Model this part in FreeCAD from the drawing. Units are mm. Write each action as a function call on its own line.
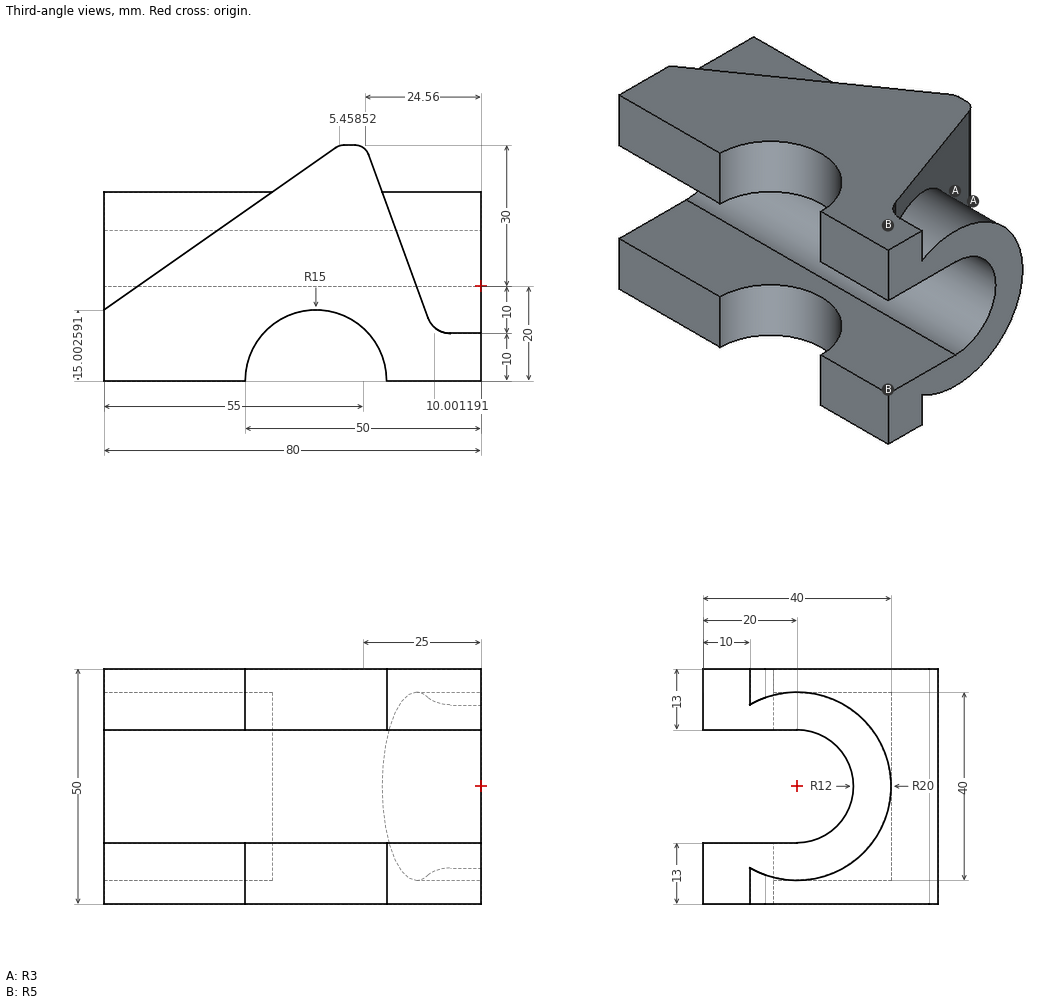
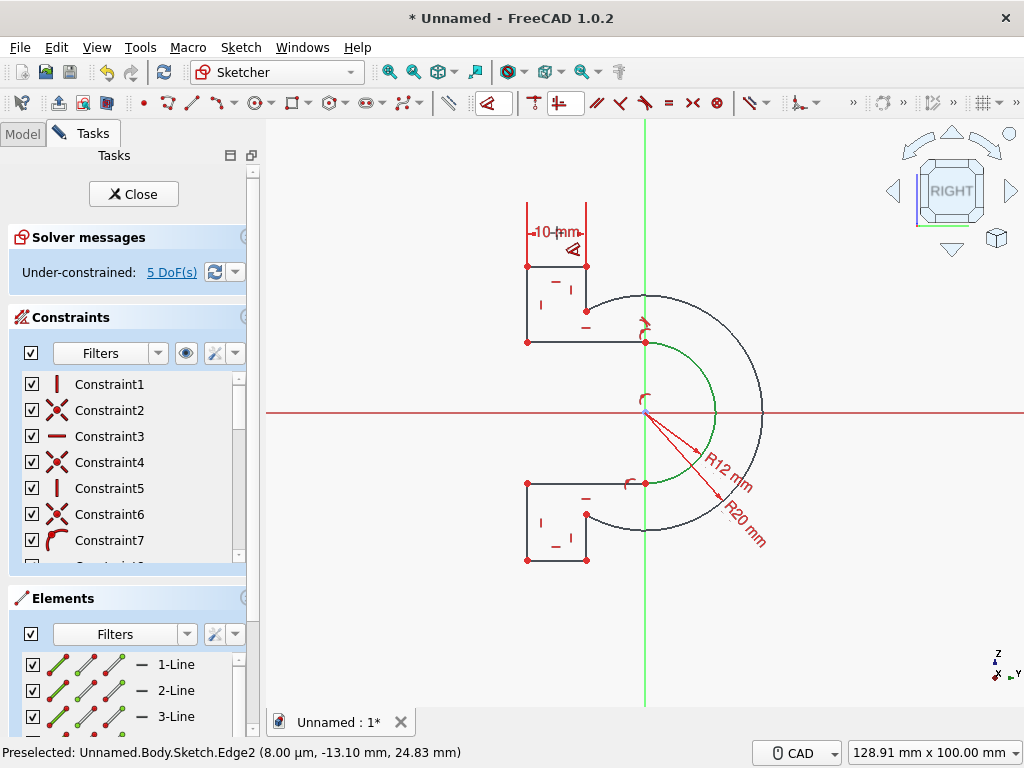
click(527, 290)
click(493, 305)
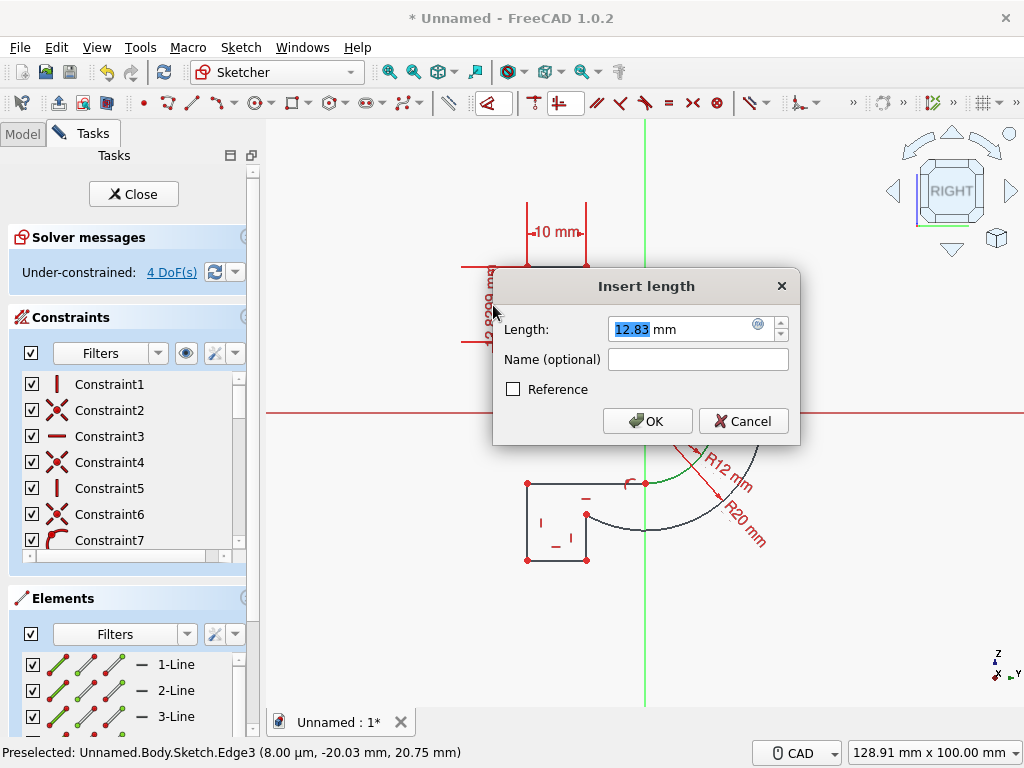
text(13)
key(Return)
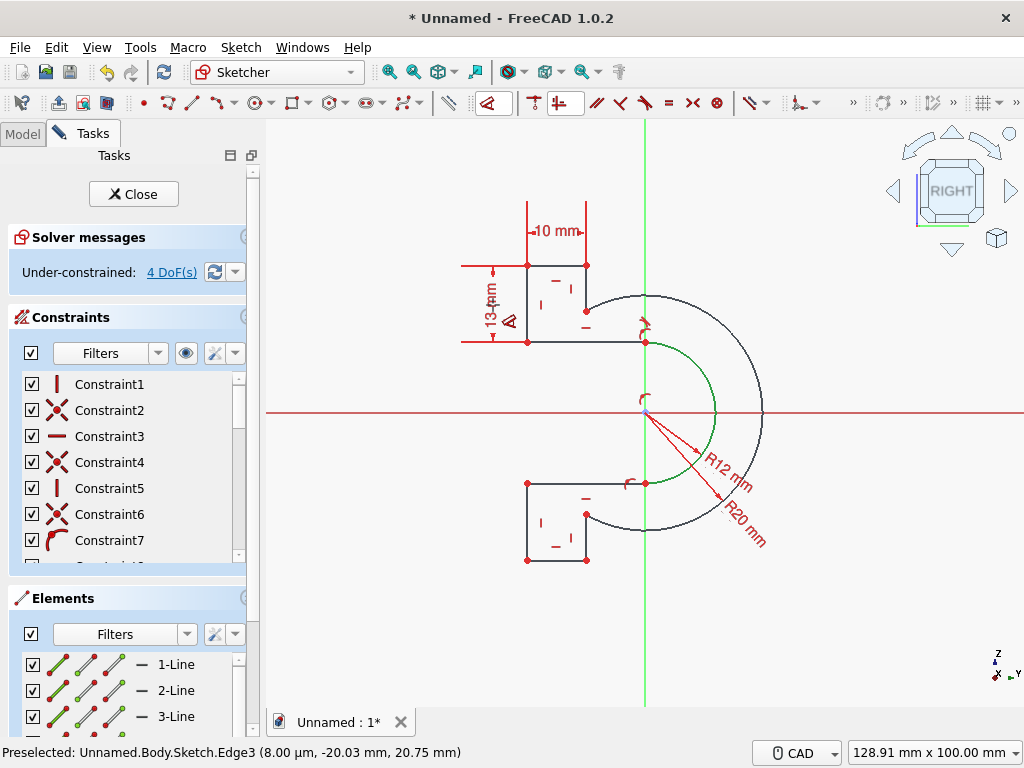
click(563, 342)
click(586, 376)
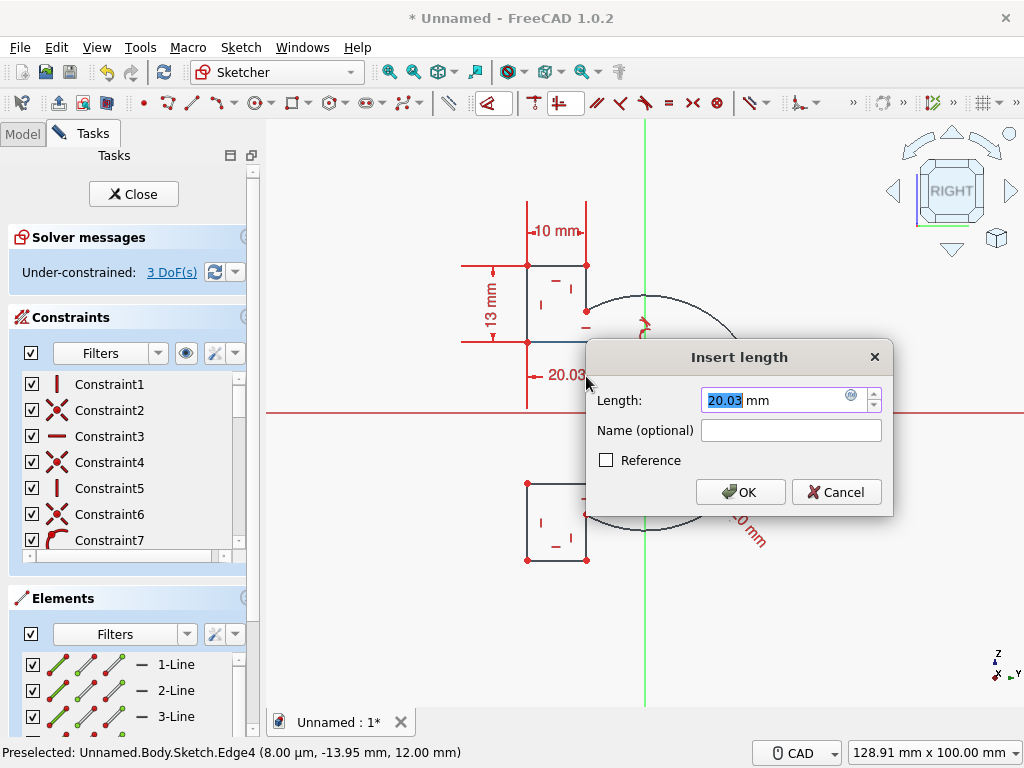
text(20)
key(Return)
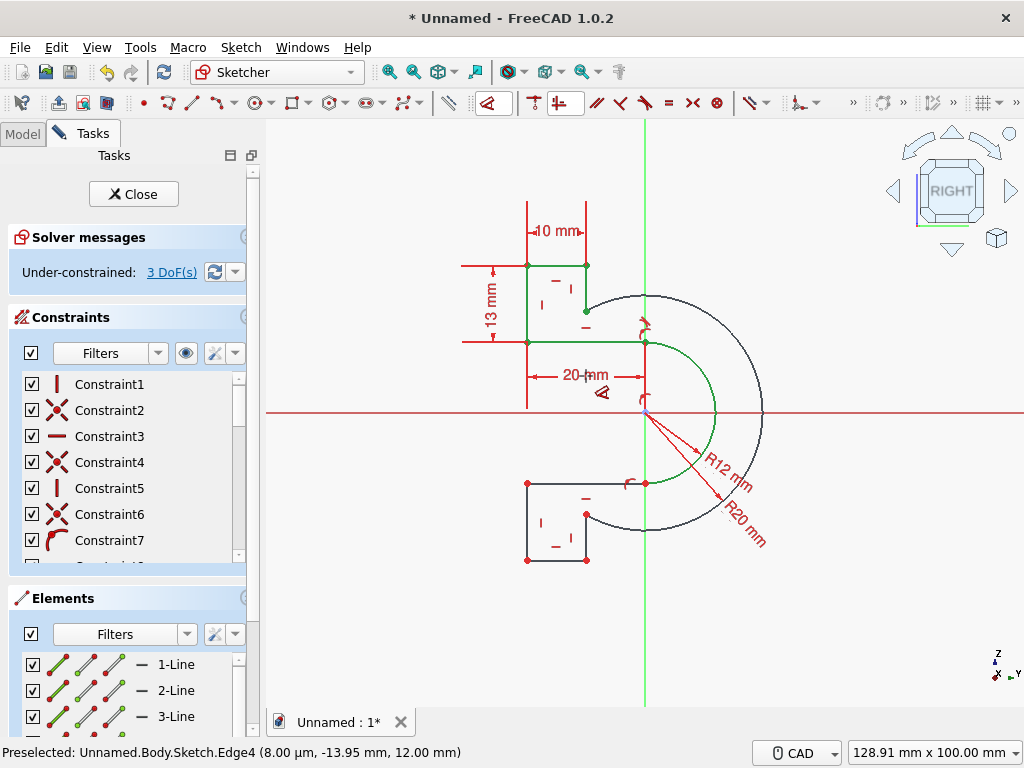
click(610, 484)
click(559, 518)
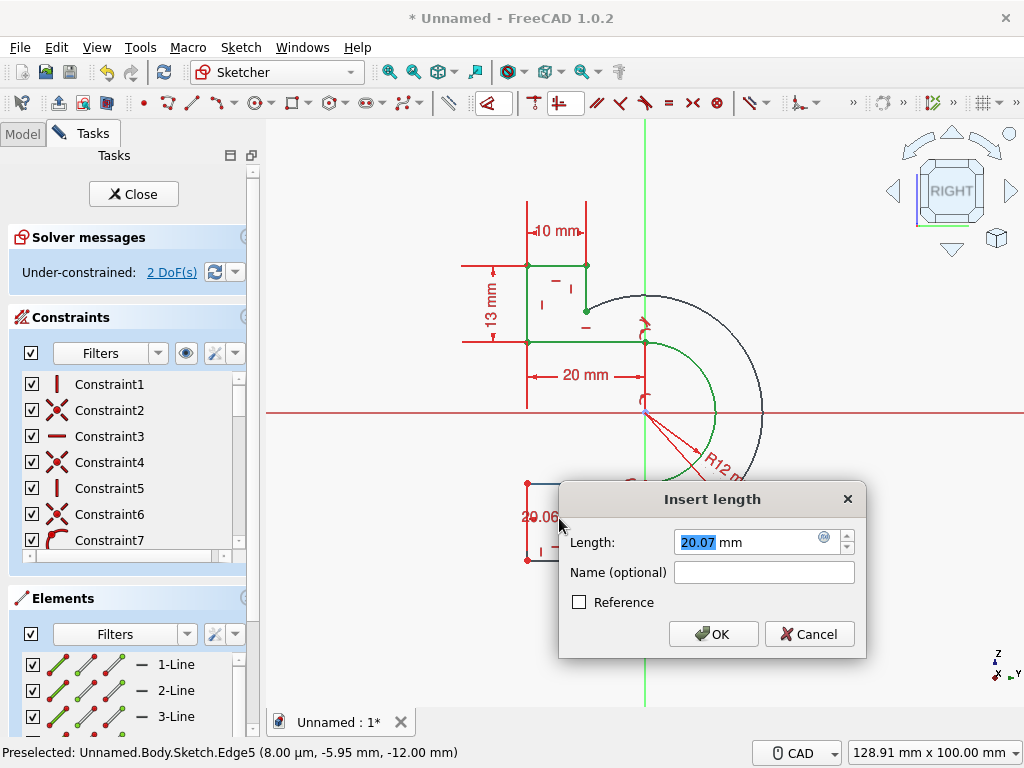
text(20)
key(Return)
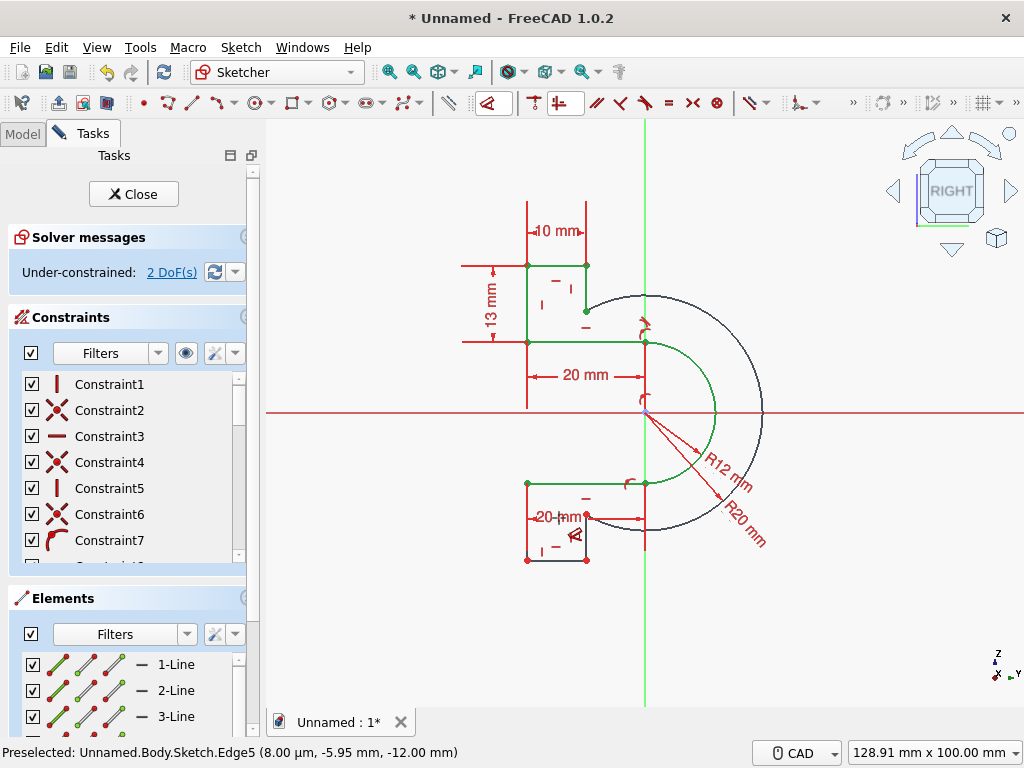
click(527, 507)
click(493, 540)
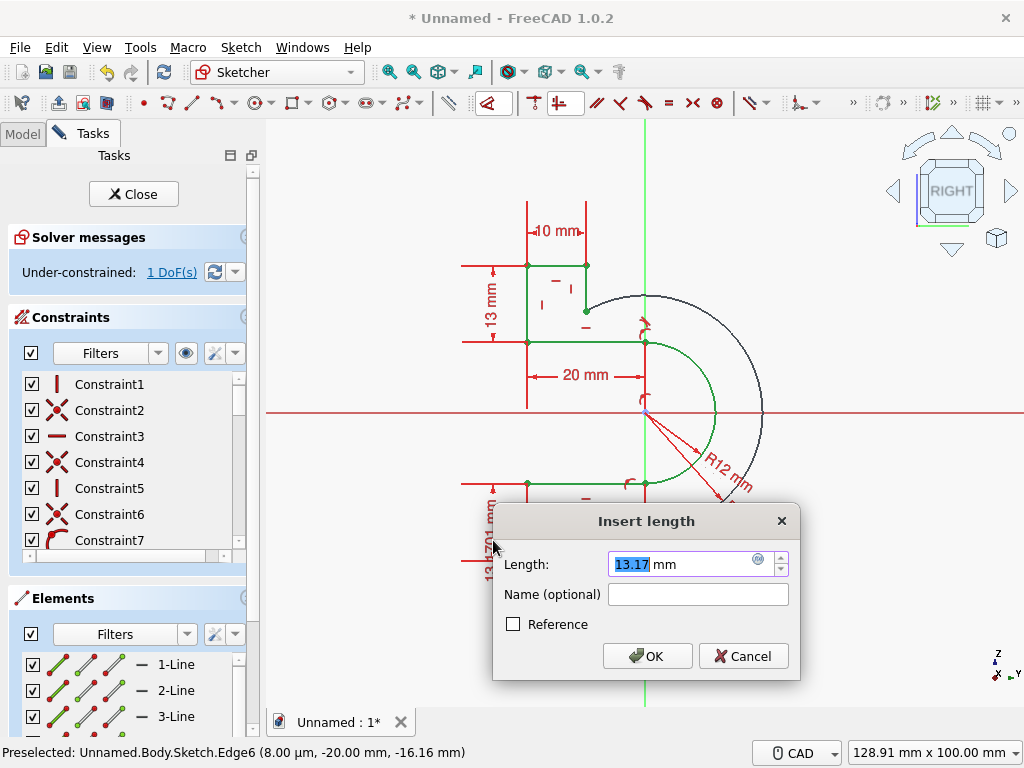
text(13)
key(Return)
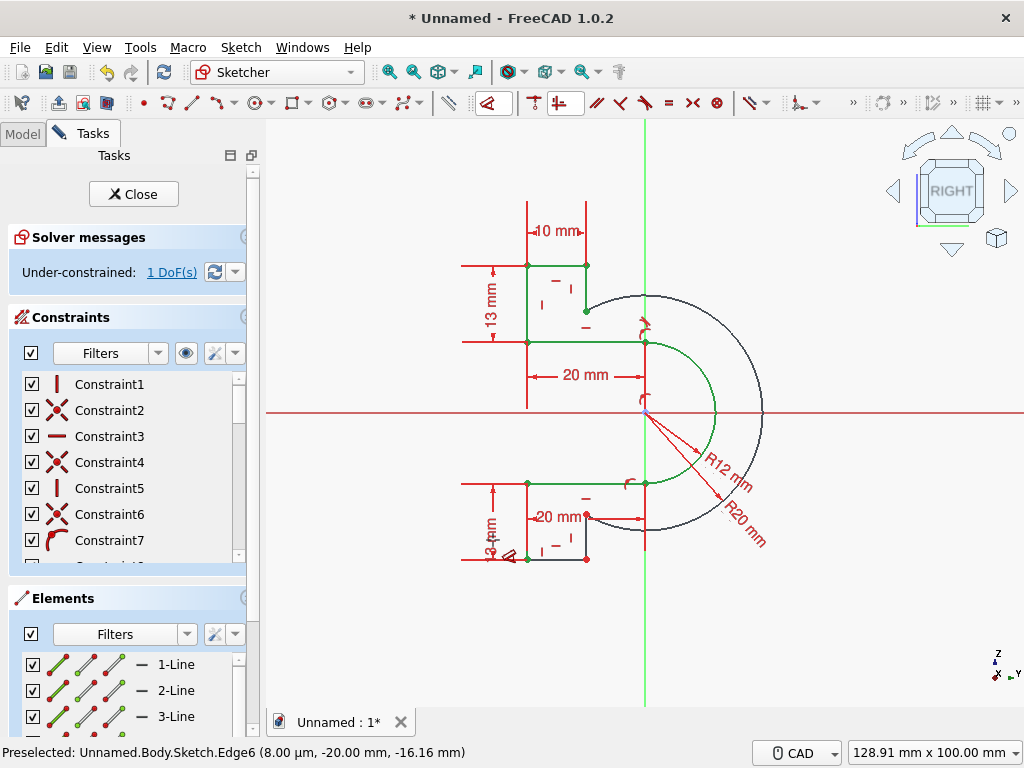
click(545, 560)
click(557, 594)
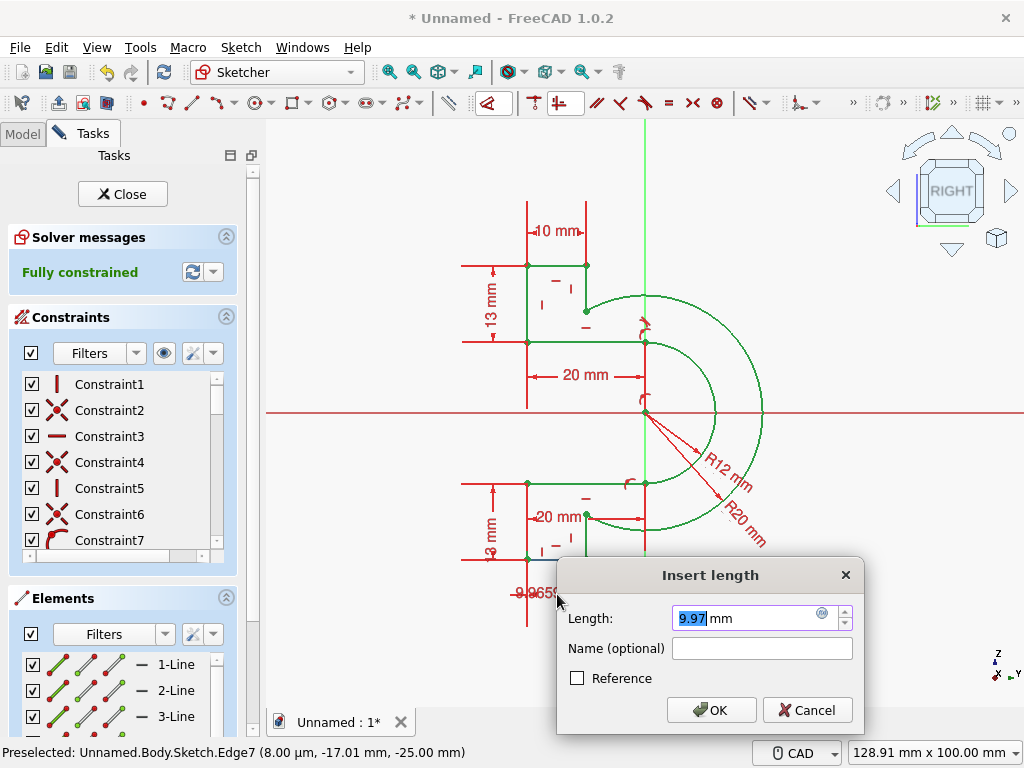
text(10)
key(Return)
key(Escape)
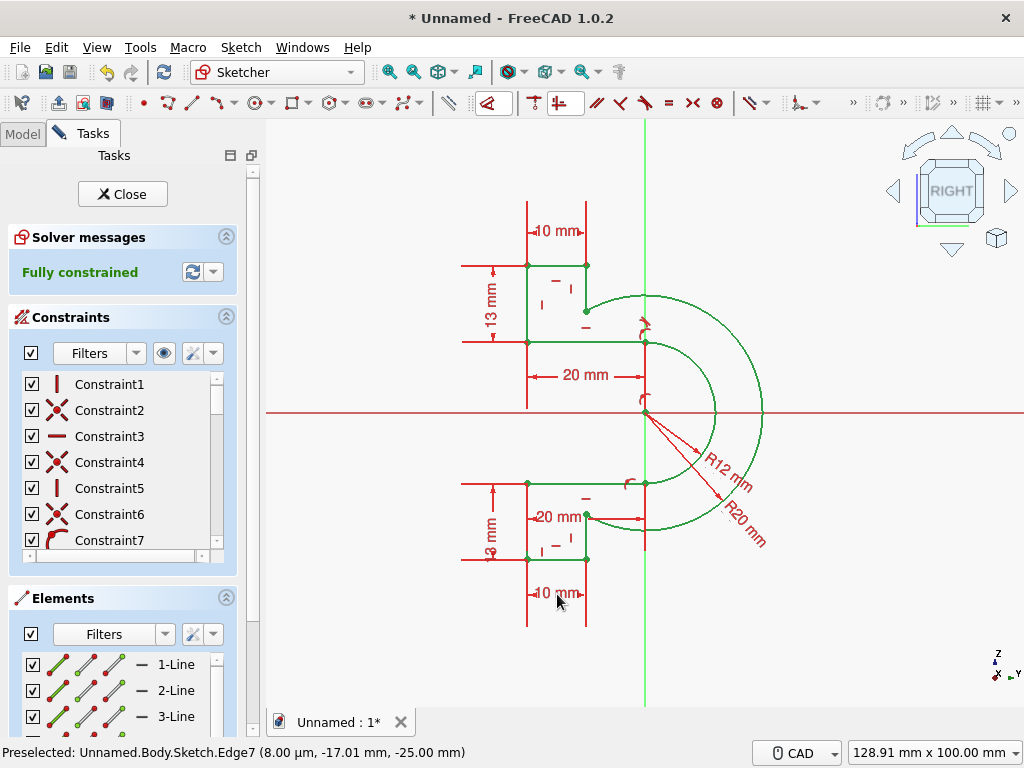
click(123, 194)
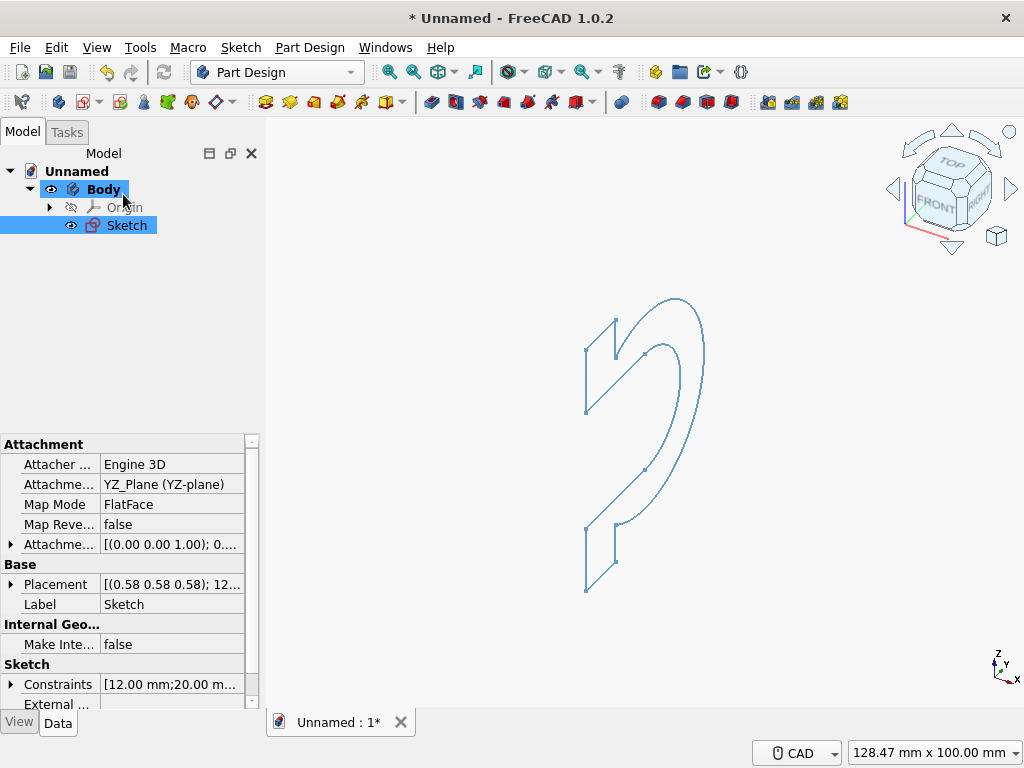
click(266, 102)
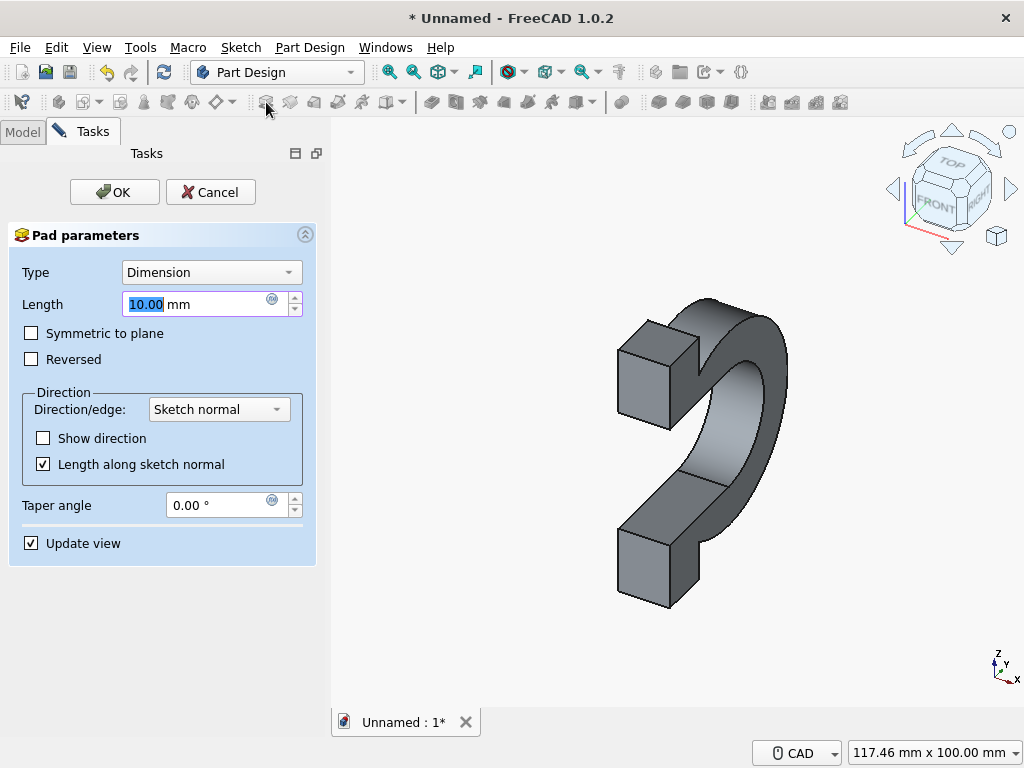
text(25)
key(Tab)